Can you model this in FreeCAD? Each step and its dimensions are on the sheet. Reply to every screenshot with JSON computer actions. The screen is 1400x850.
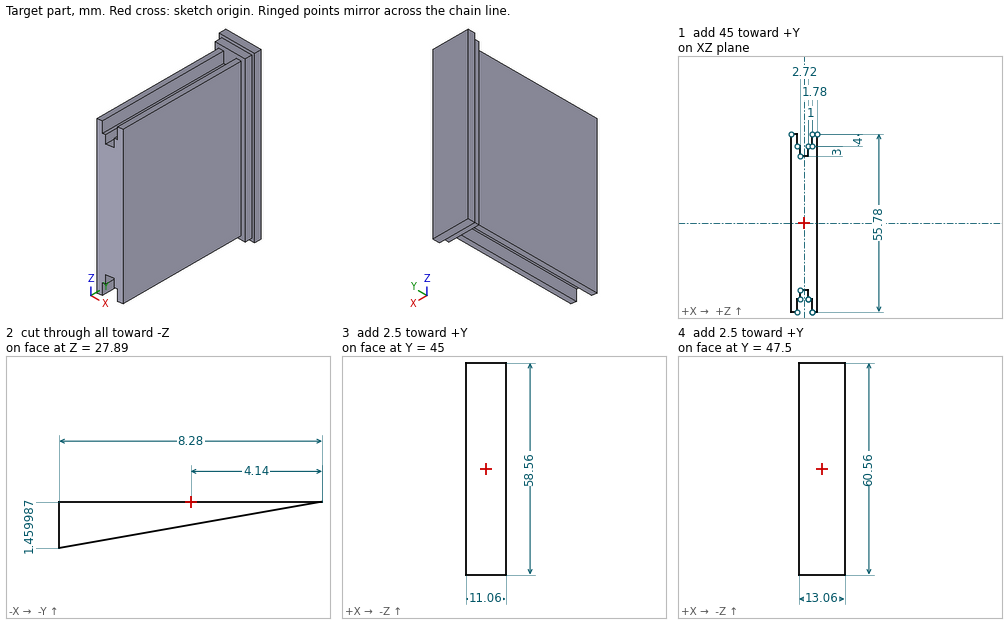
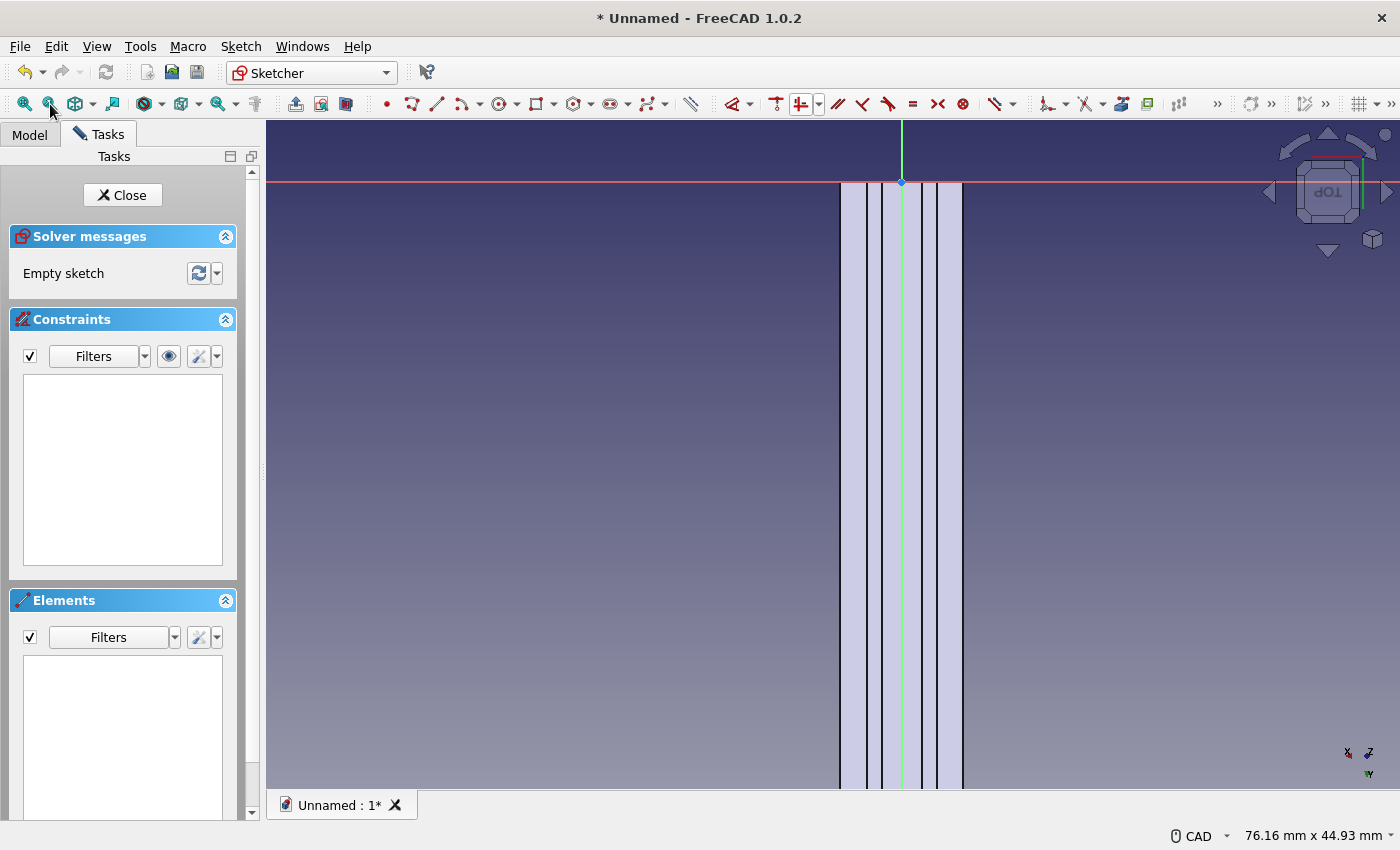
{"action": "scroll", "coordinate": [936, 148], "scroll_direction": "up", "scroll_amount": 8}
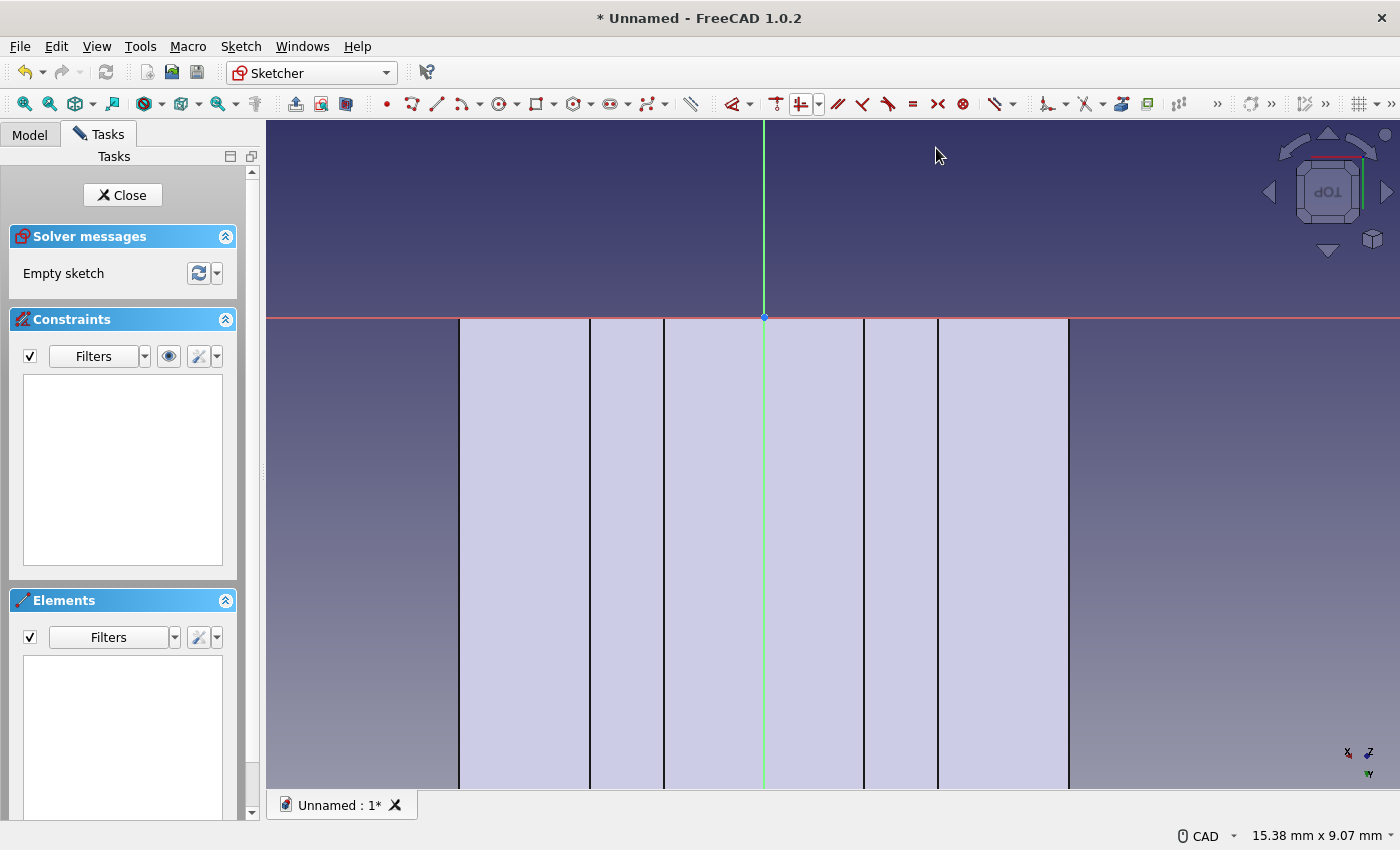
{"action": "key", "text": "g m"}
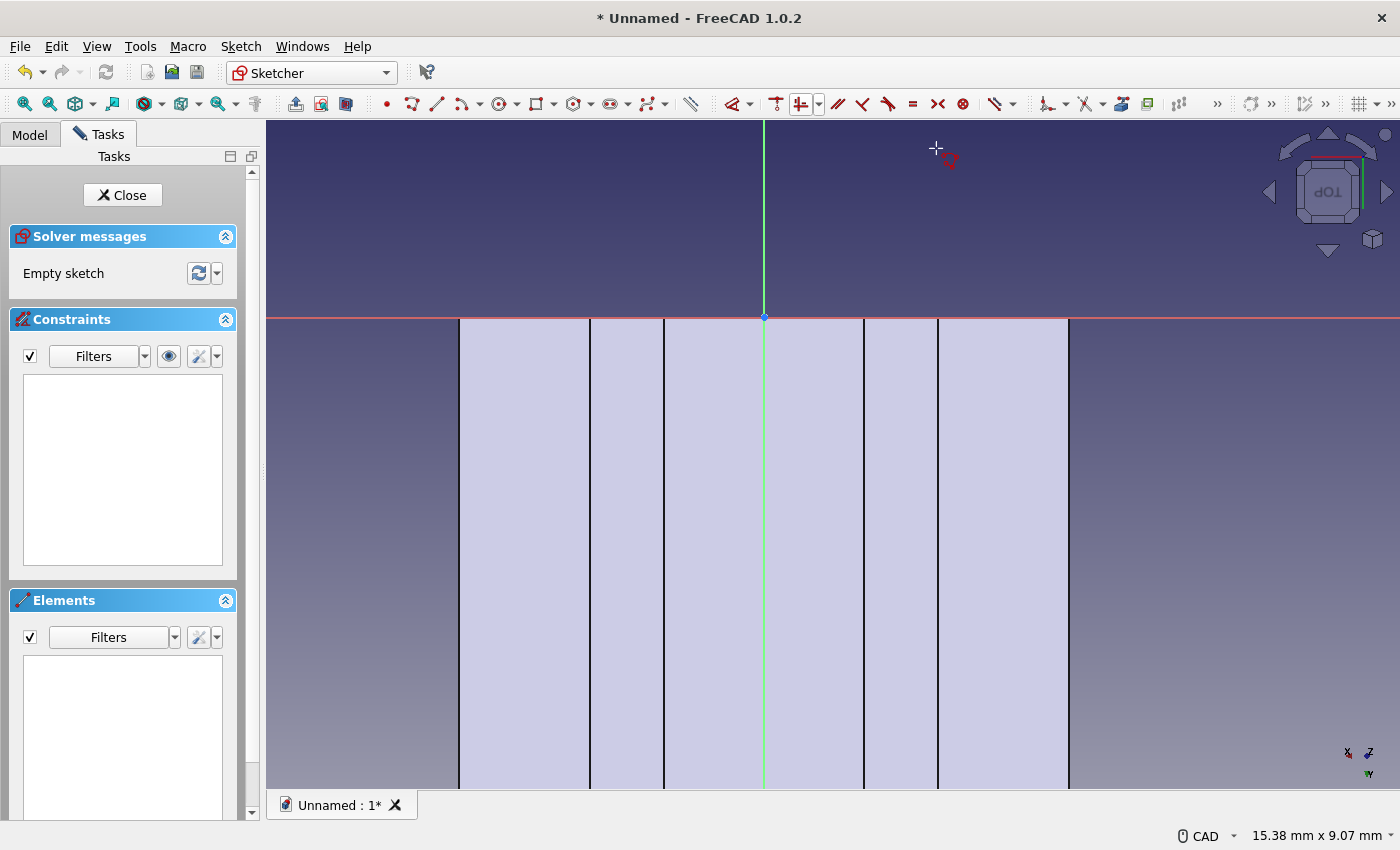
{"action": "left_click", "coordinate": [1069, 318]}
{"action": "left_click", "coordinate": [459, 327]}
{"action": "left_click", "coordinate": [459, 425]}
{"action": "left_click", "coordinate": [1069, 318]}
{"action": "key", "text": "Escape"}
{"action": "key", "text": "Escape"}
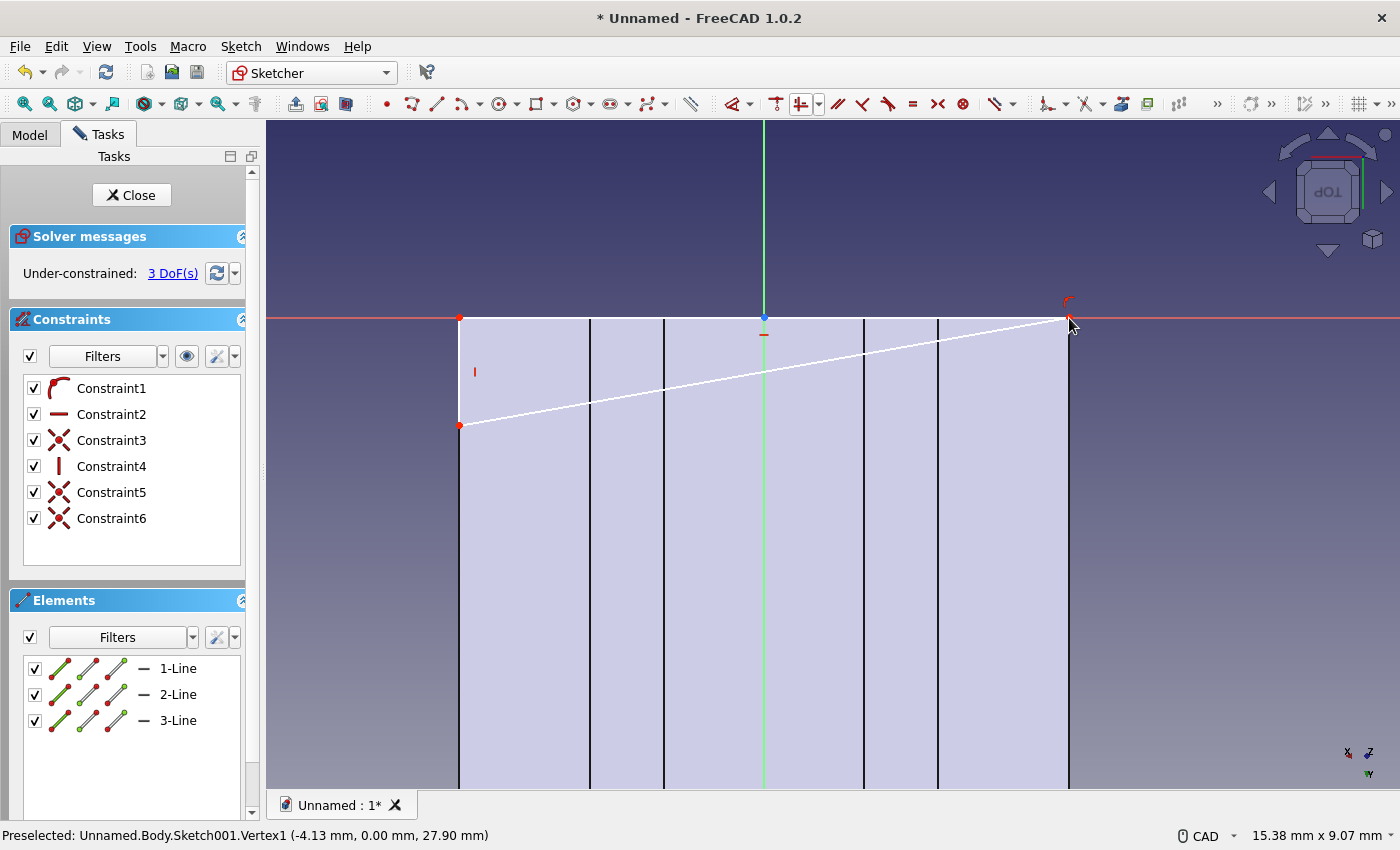
{"action": "key", "text": "d"}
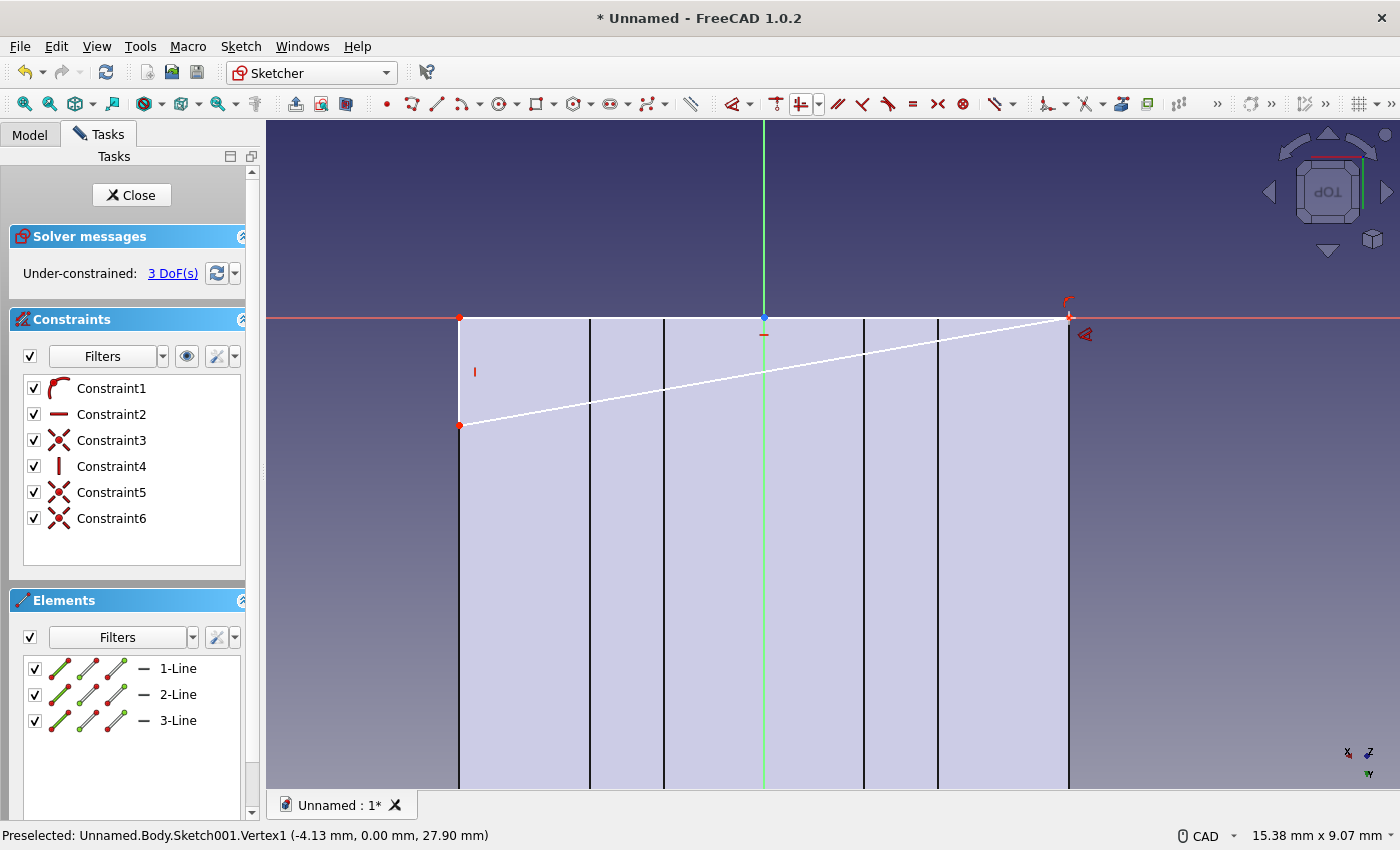
{"action": "left_click", "coordinate": [886, 318]}
{"action": "left_click", "coordinate": [624, 284]}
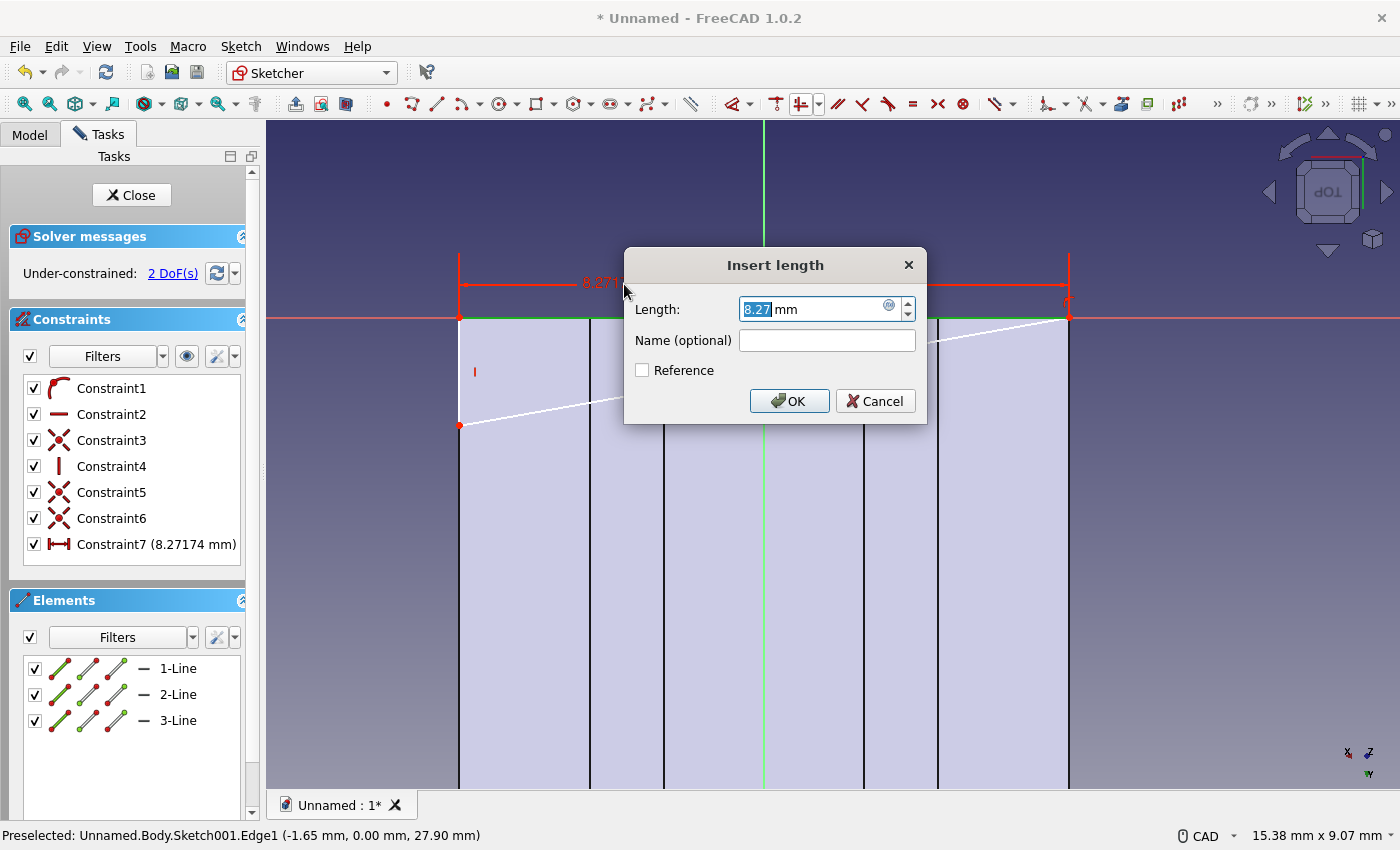
{"action": "type", "text": "8.28"}
{"action": "key", "text": "Return"}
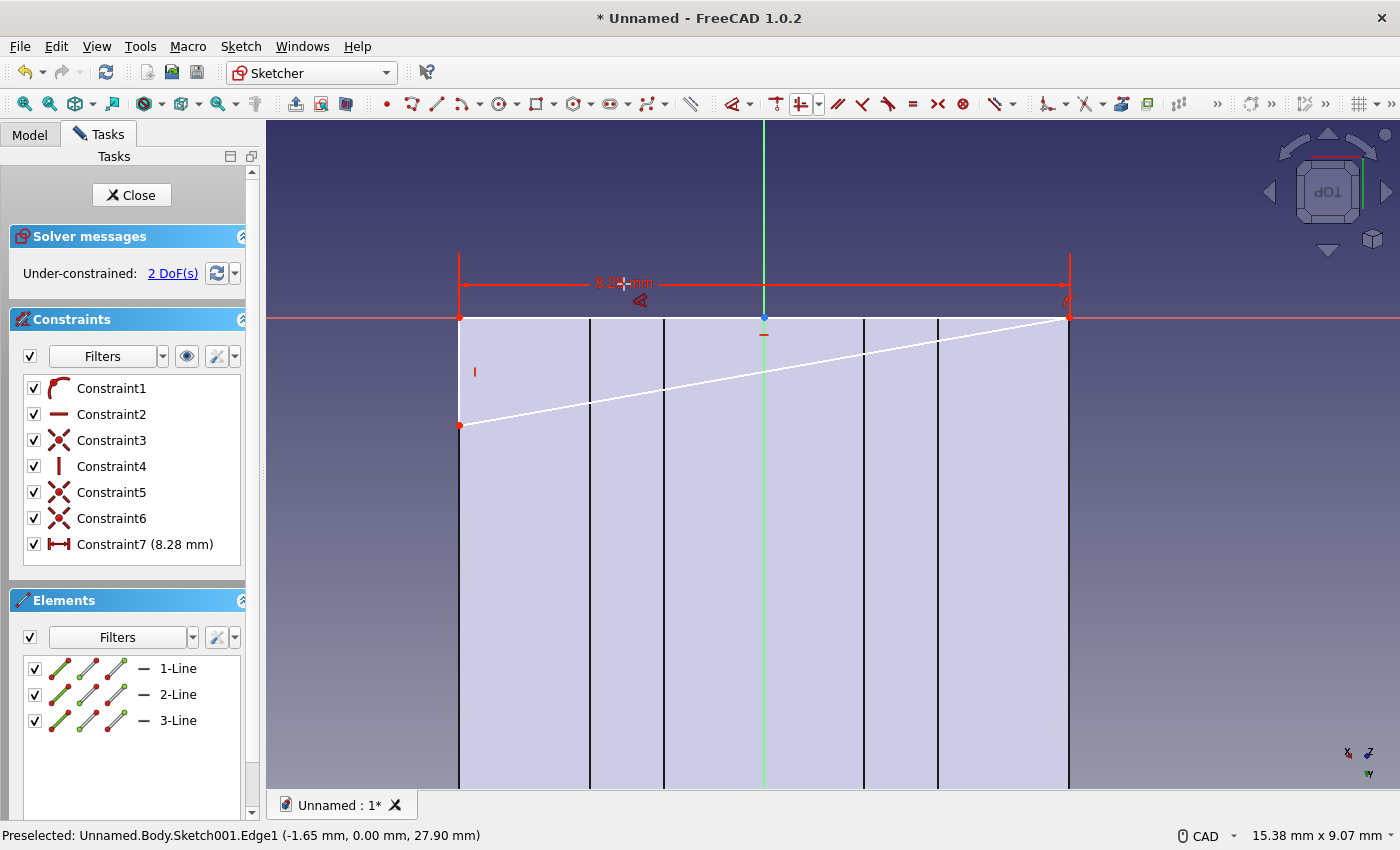
{"action": "left_click", "coordinate": [1070, 318]}
{"action": "left_click", "coordinate": [917, 284]}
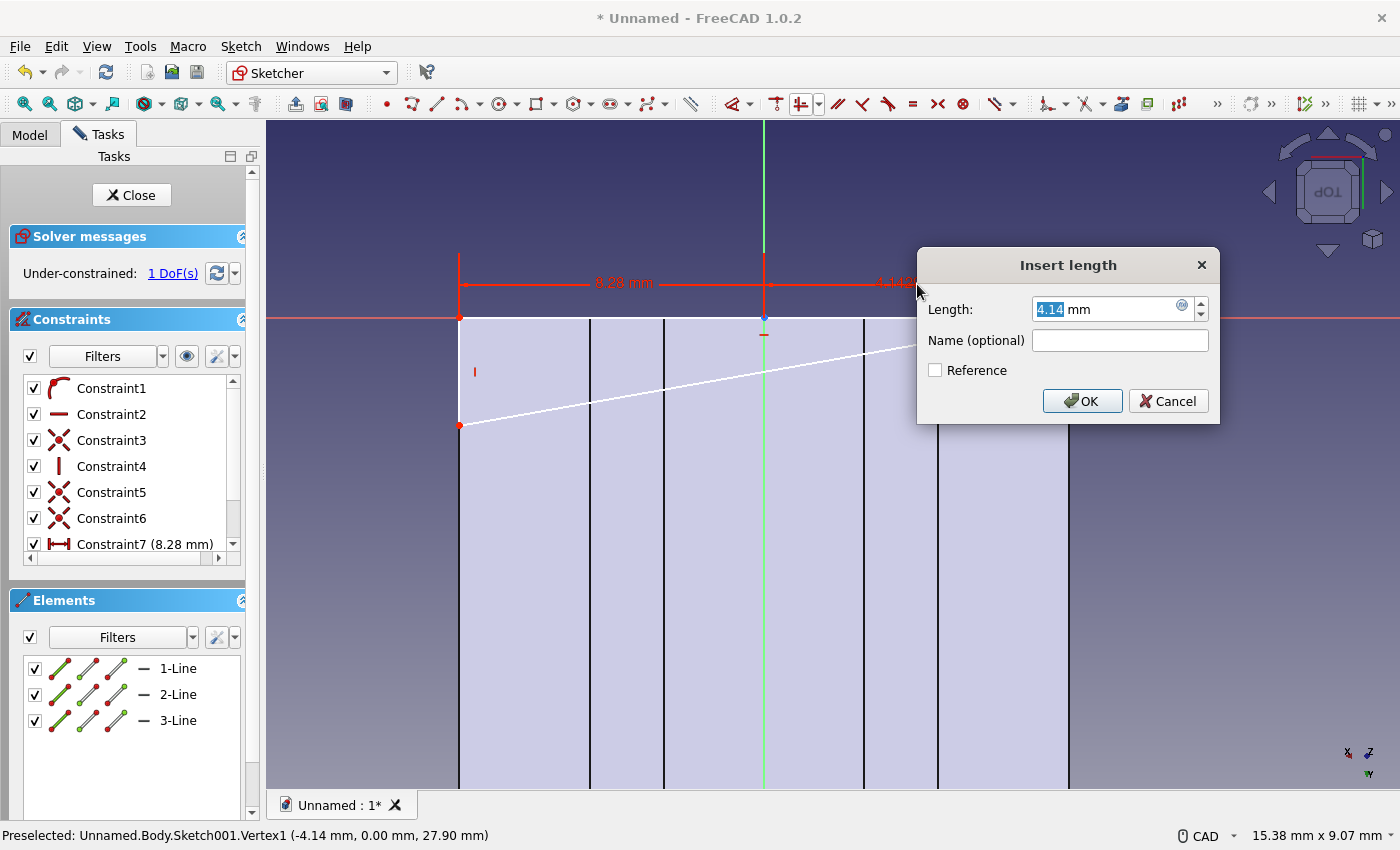
{"action": "type", "text": "4.14"}
{"action": "key", "text": "Return"}